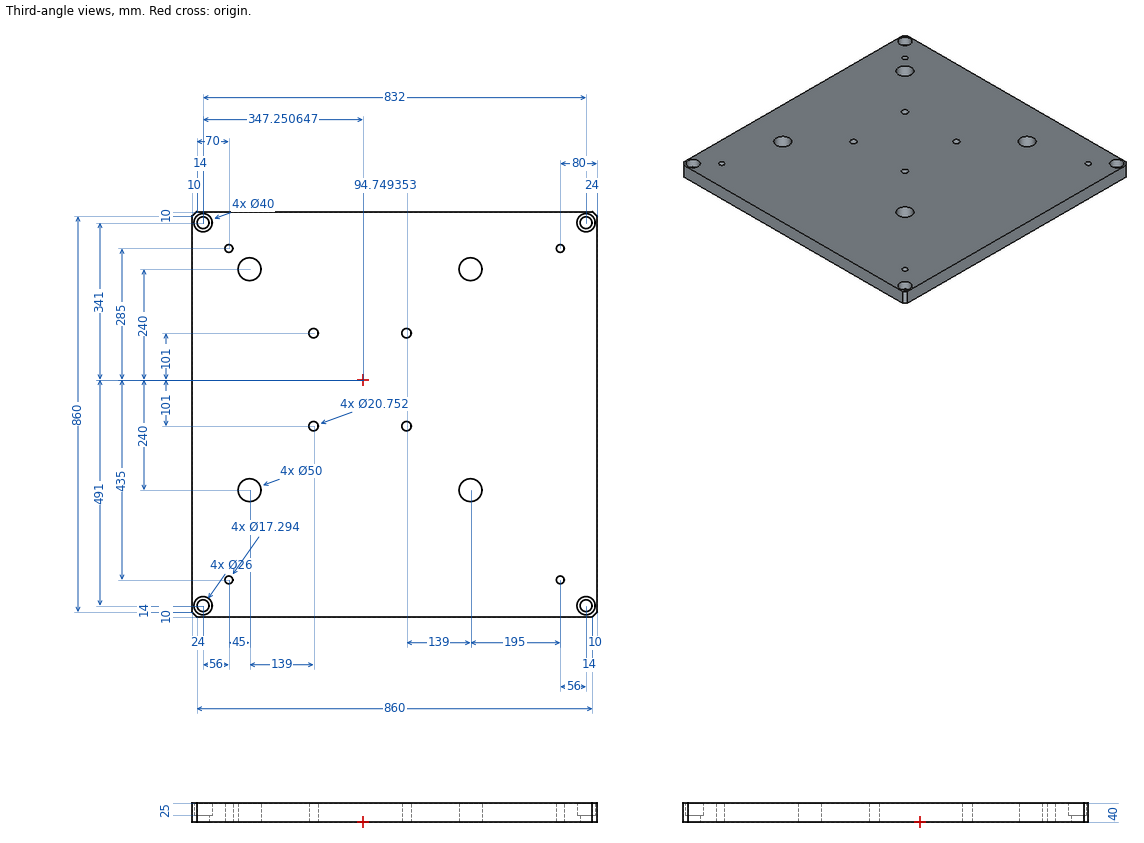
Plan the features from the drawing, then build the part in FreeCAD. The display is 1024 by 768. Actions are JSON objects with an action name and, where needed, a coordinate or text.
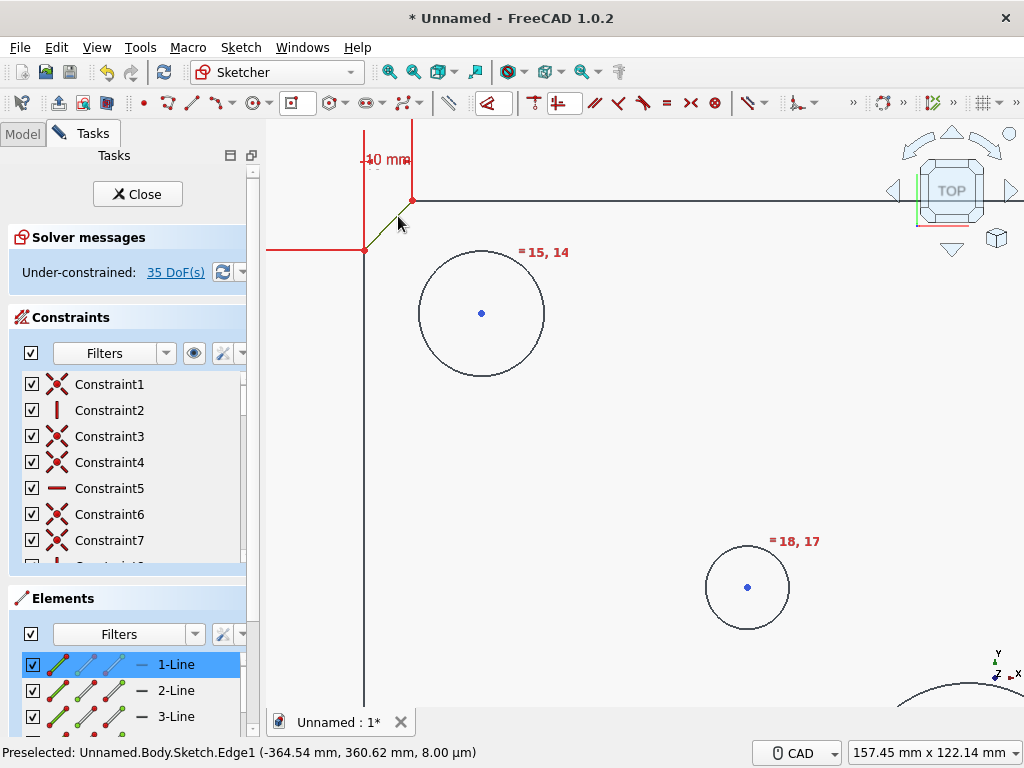
{"action": "left_click", "coordinate": [506, 104]}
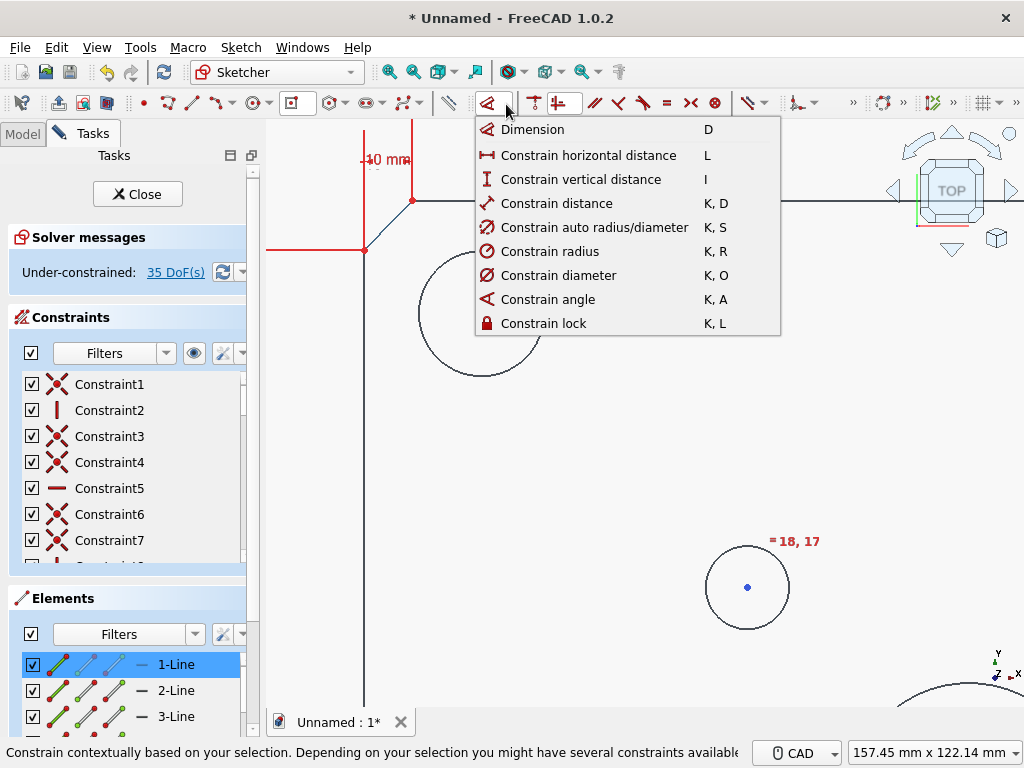
{"action": "left_click", "coordinate": [628, 179]}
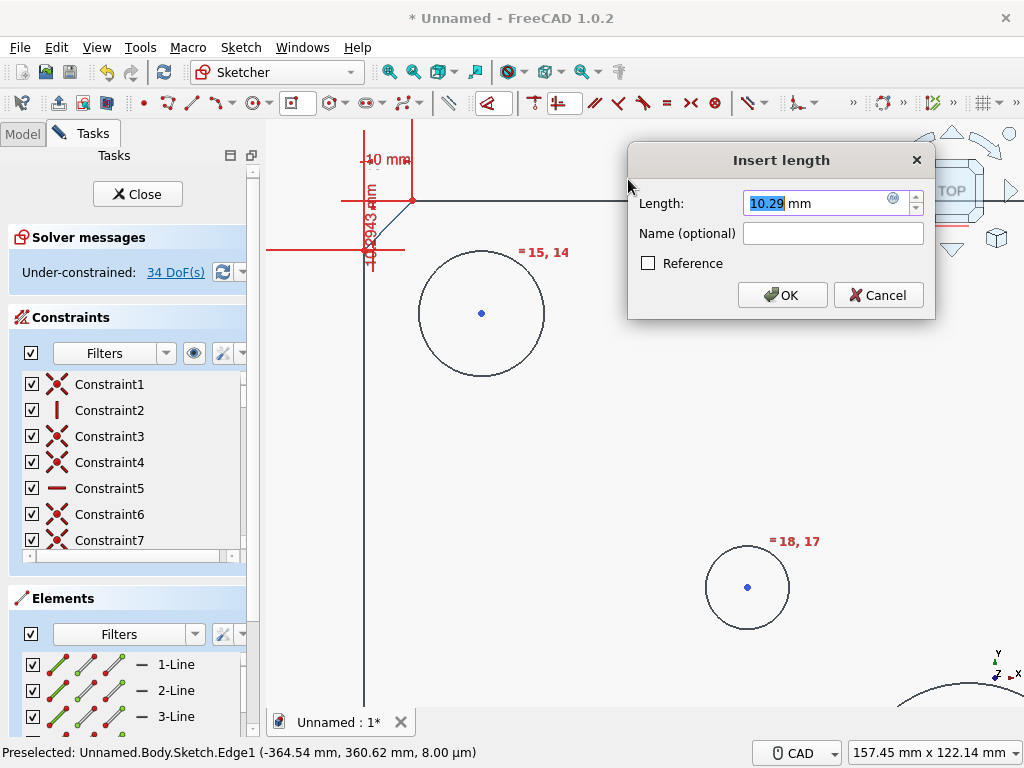
{"action": "type", "text": "10"}
{"action": "key", "text": "Return"}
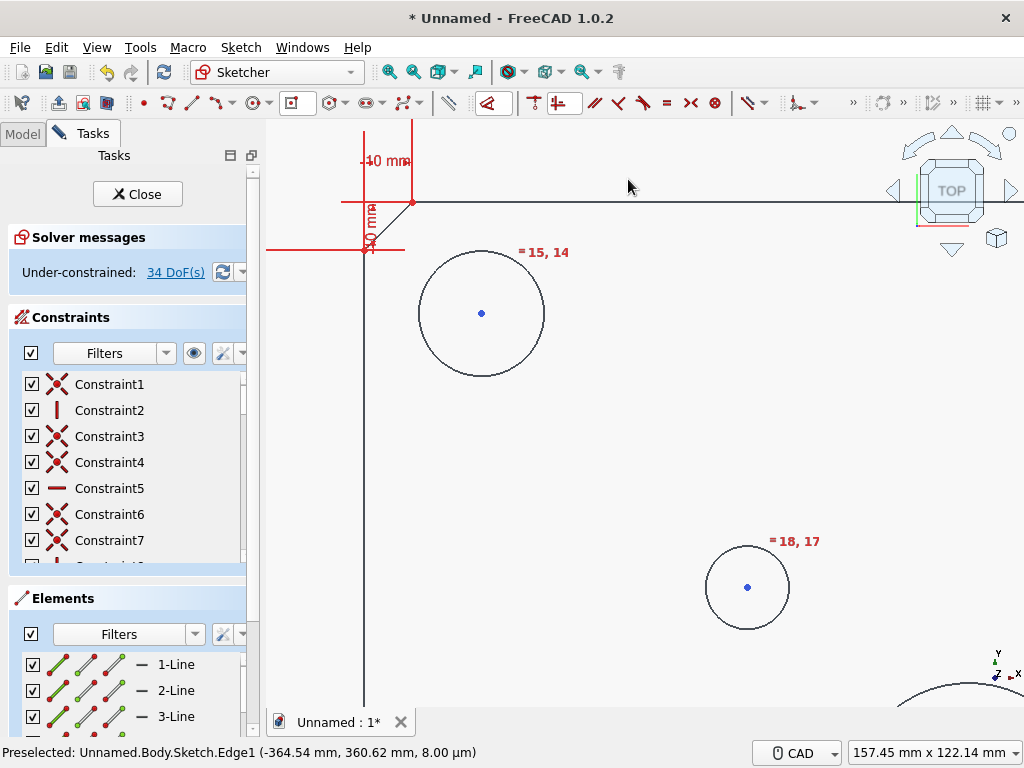
{"action": "scroll", "coordinate": [386, 223], "scroll_direction": "down", "scroll_amount": 12}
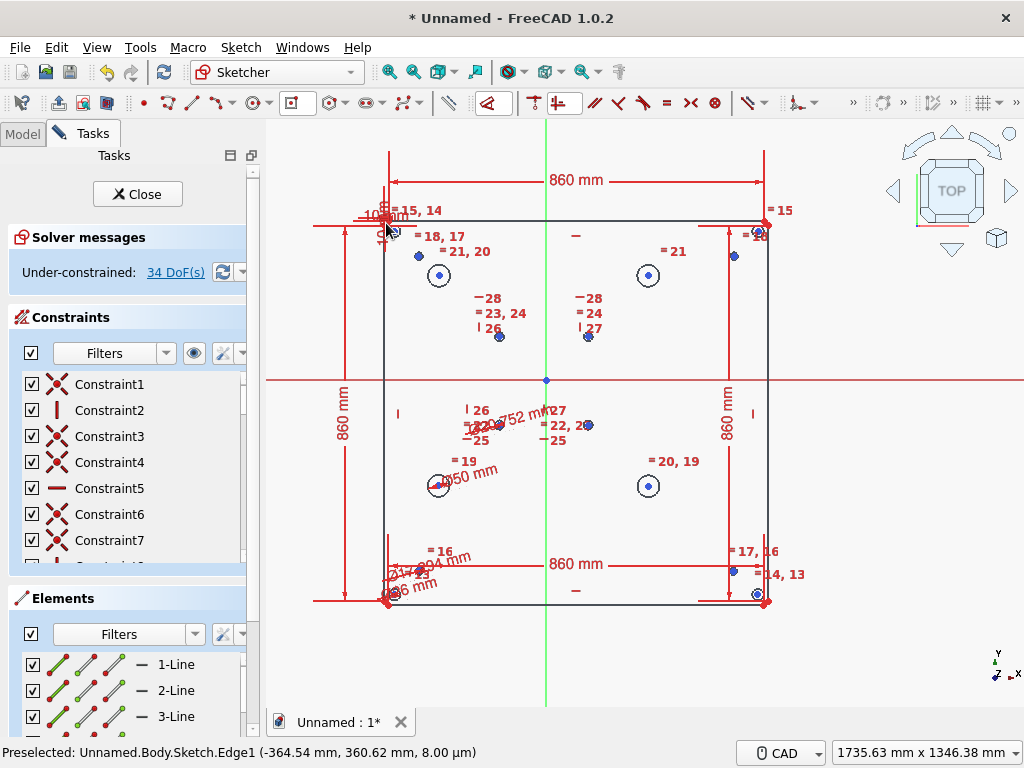
{"action": "scroll", "coordinate": [385, 602], "scroll_direction": "up", "scroll_amount": 12}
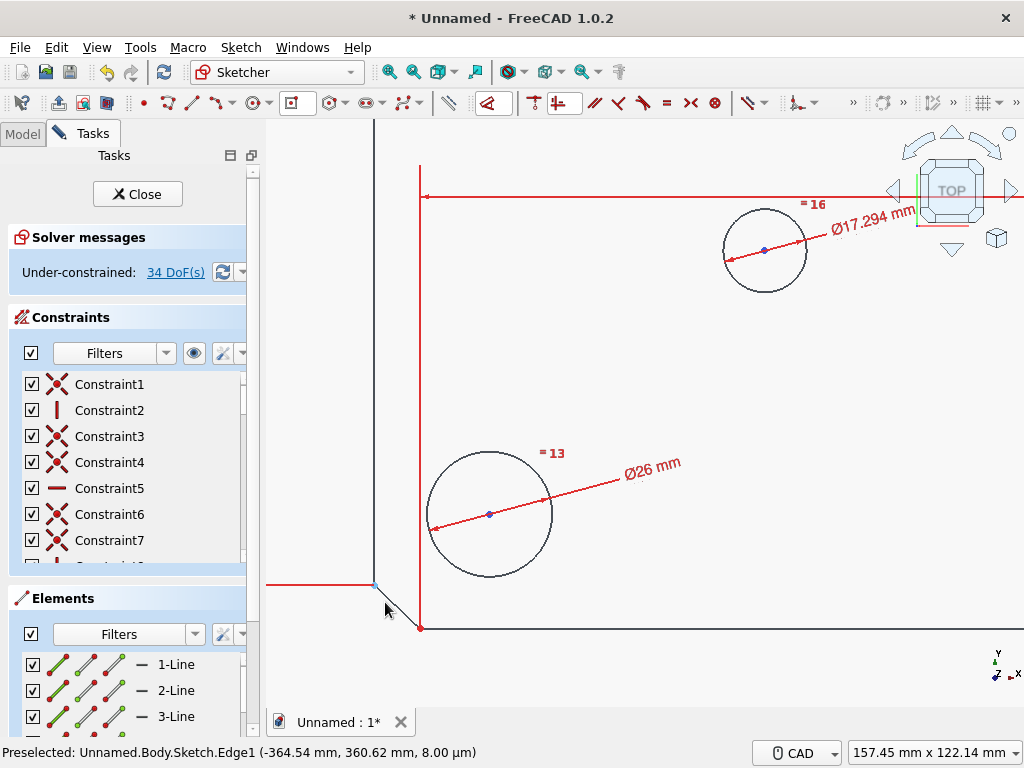
{"action": "left_click", "coordinate": [388, 598]}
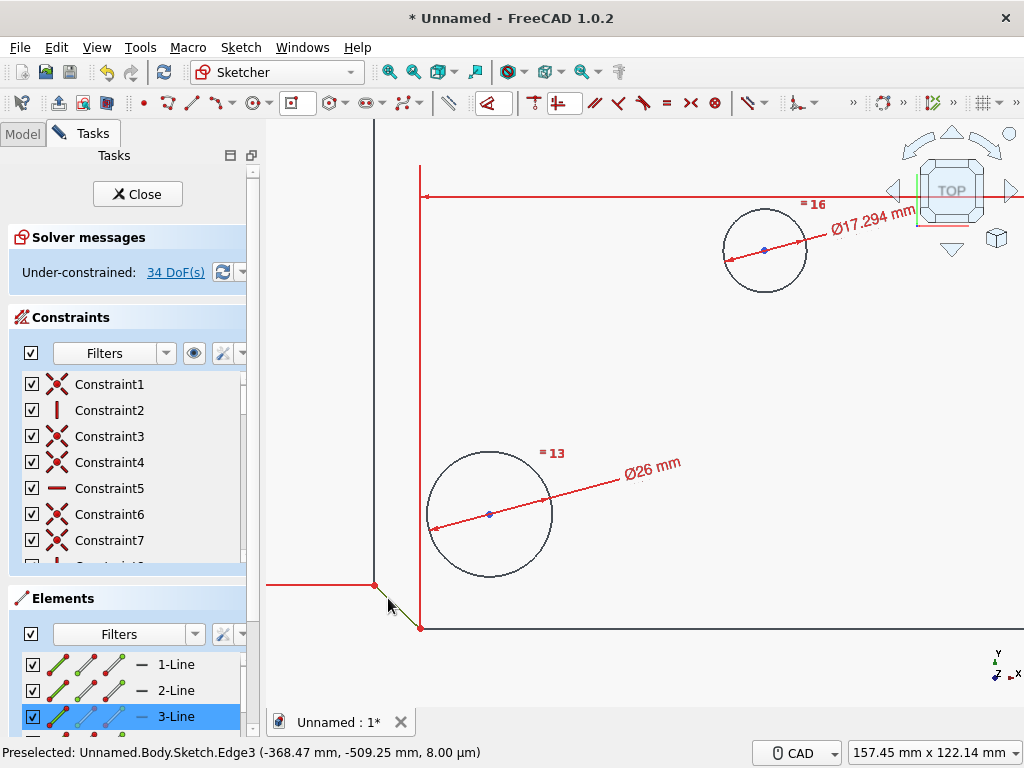
{"action": "key", "text": "l"}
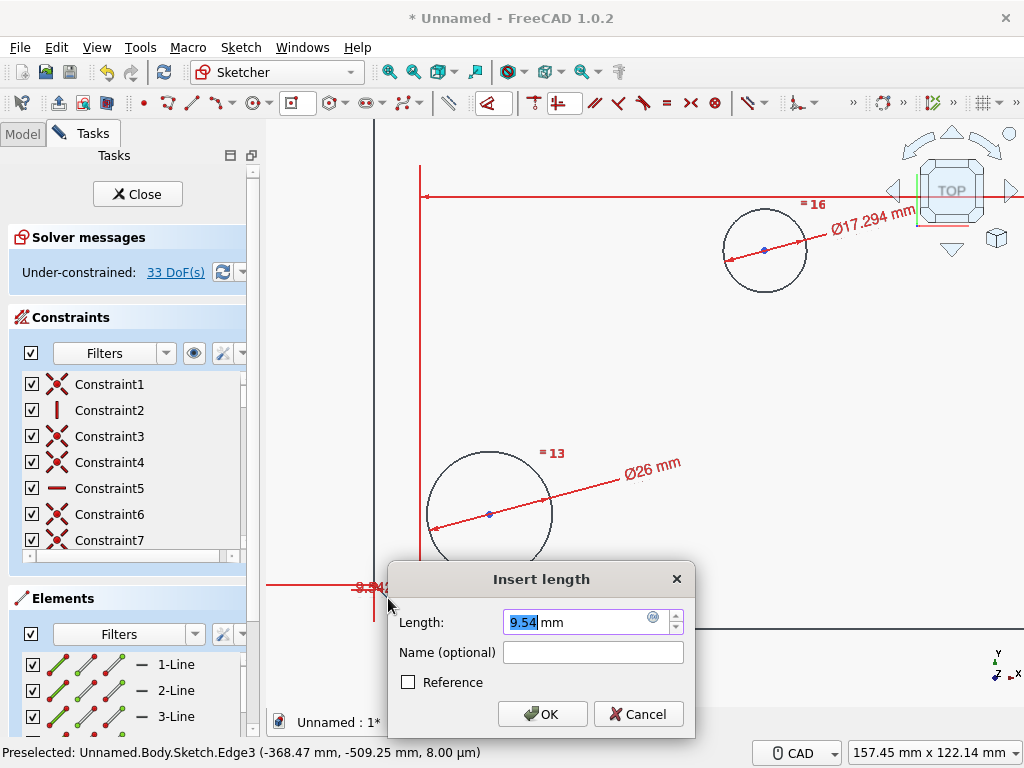
{"action": "type", "text": "10"}
{"action": "key", "text": "Return"}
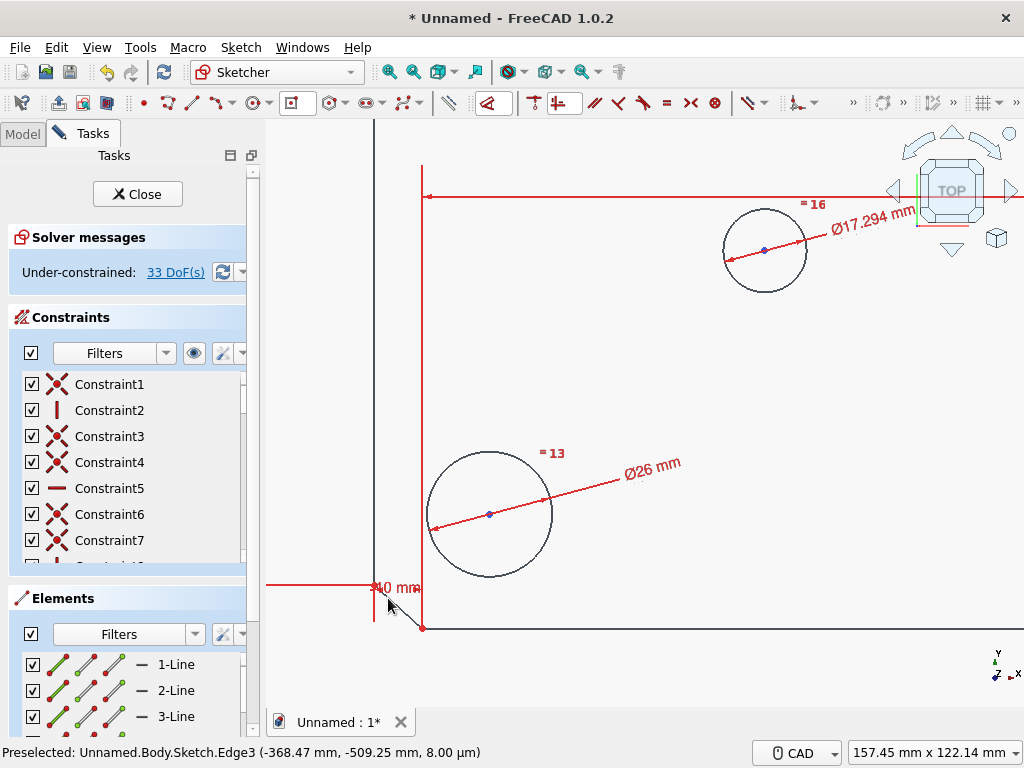
{"action": "left_click", "coordinate": [389, 598]}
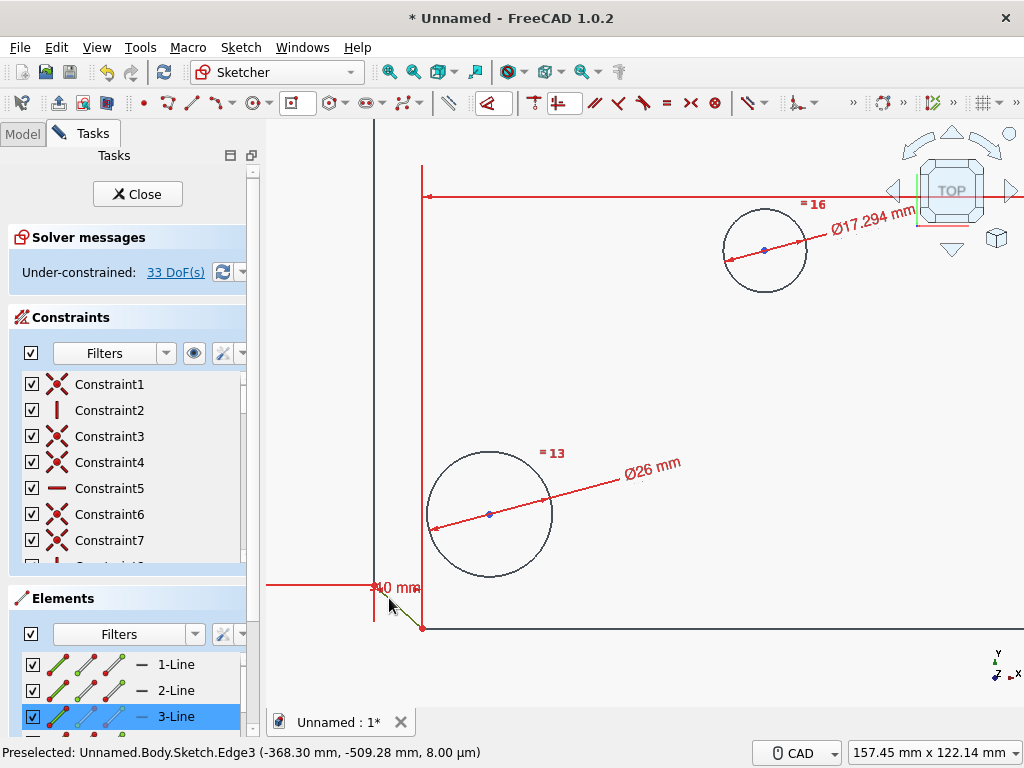
{"action": "left_click", "coordinate": [506, 104]}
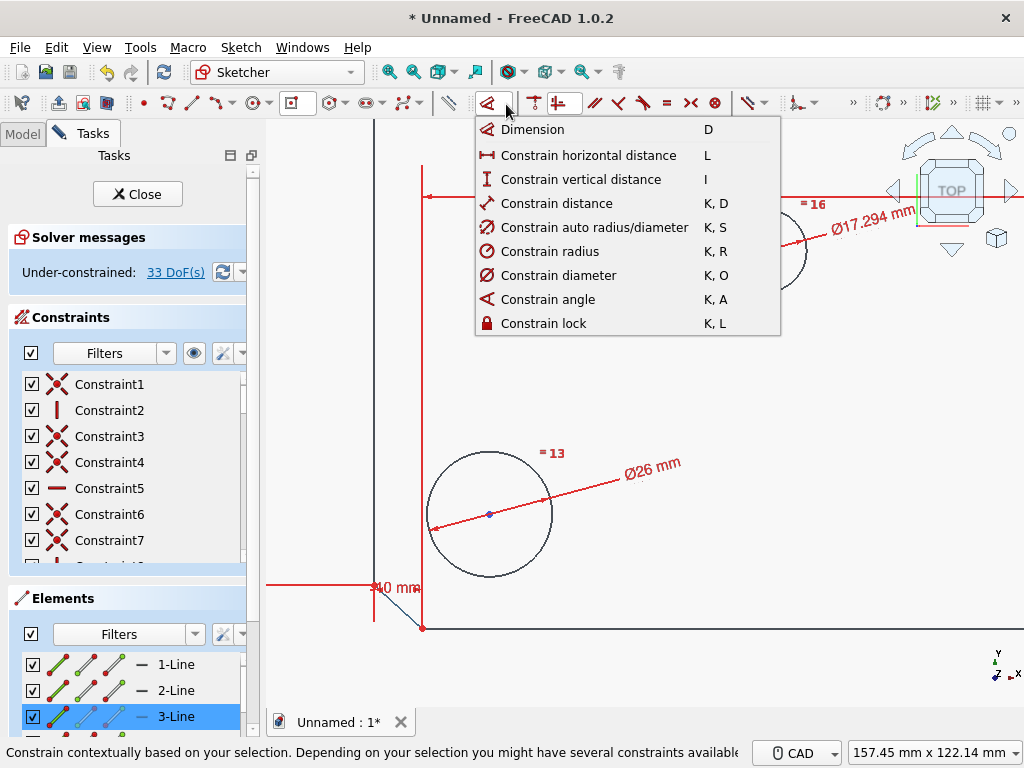
{"action": "left_click", "coordinate": [628, 179]}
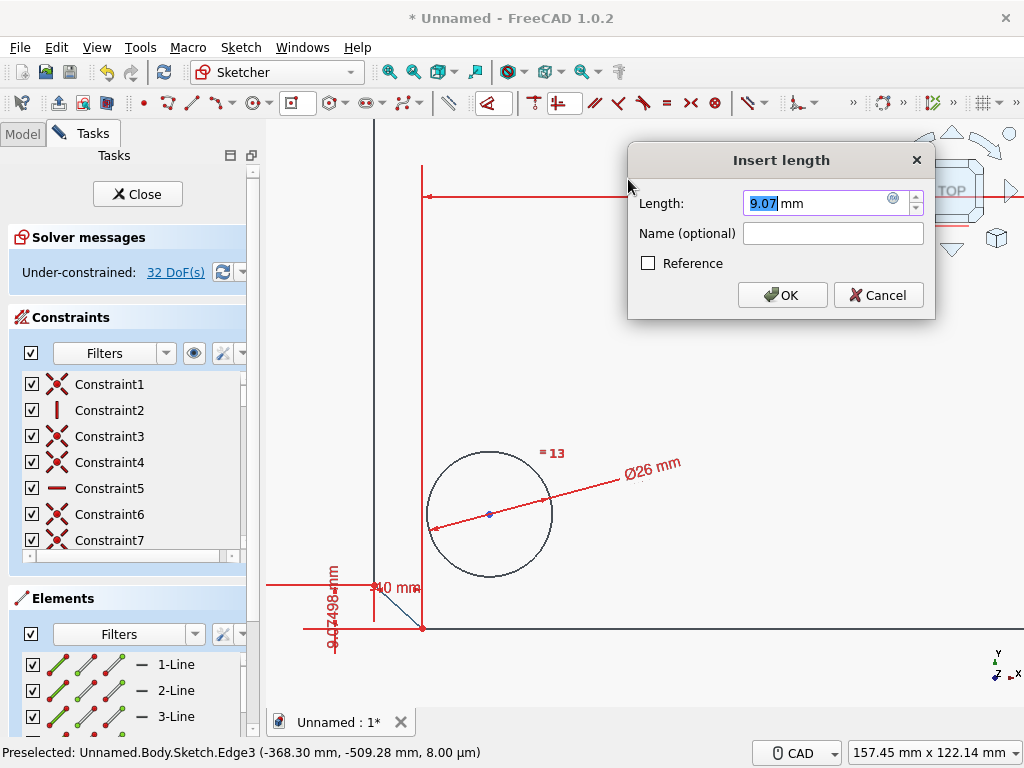
{"action": "type", "text": "10"}
{"action": "key", "text": "Return"}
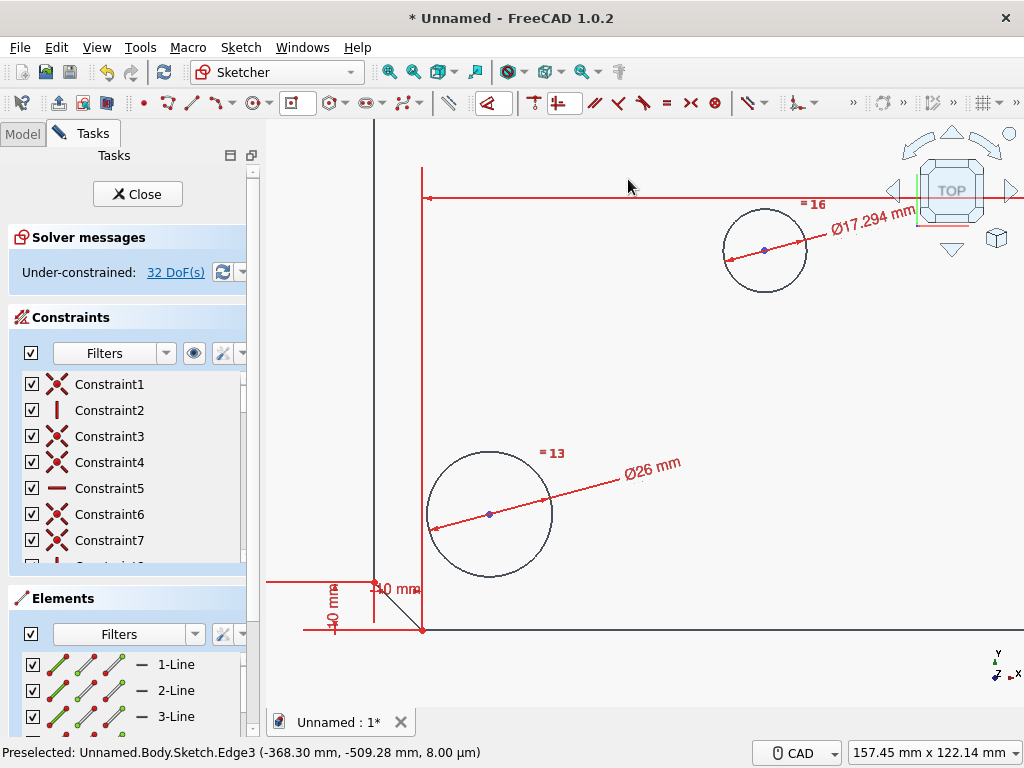
{"action": "scroll", "coordinate": [385, 603], "scroll_direction": "down", "scroll_amount": 12}